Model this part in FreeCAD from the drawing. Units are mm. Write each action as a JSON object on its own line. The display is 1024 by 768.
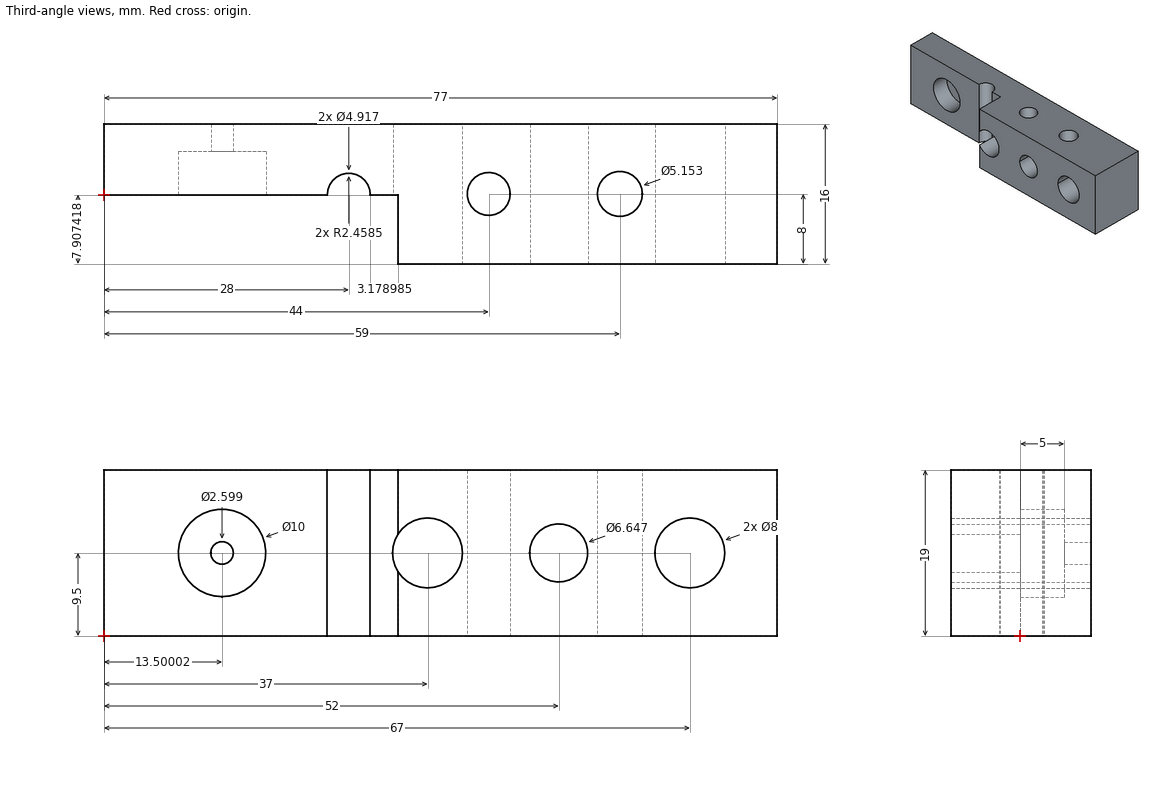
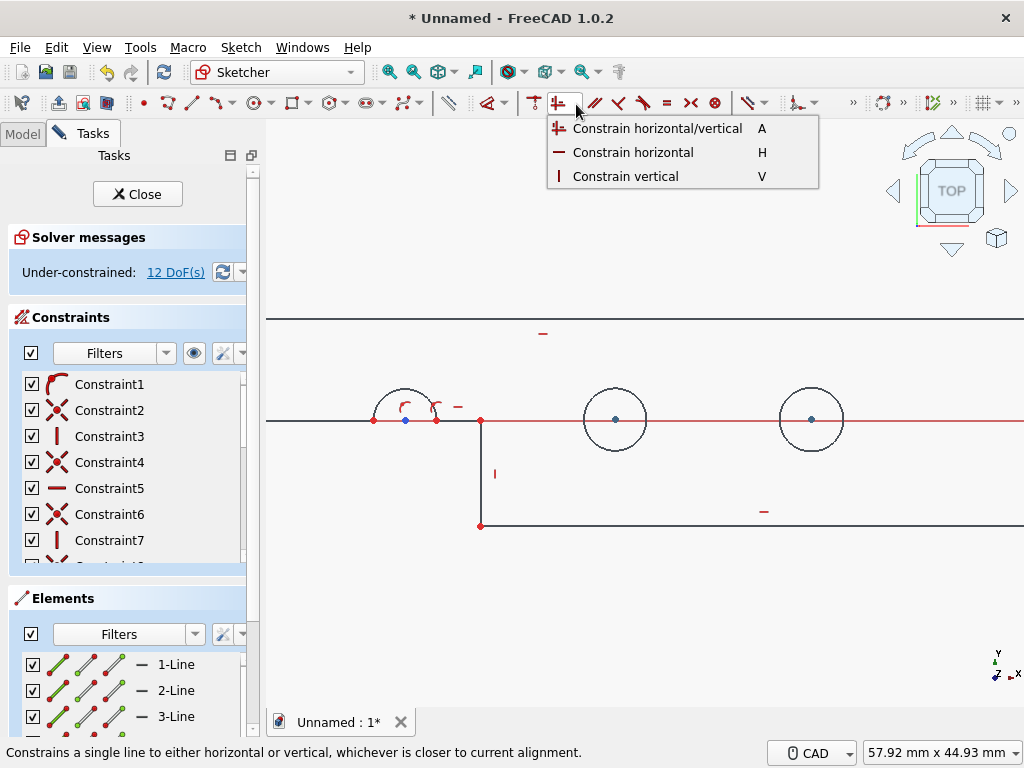
{"action": "left_click", "coordinate": [683, 152]}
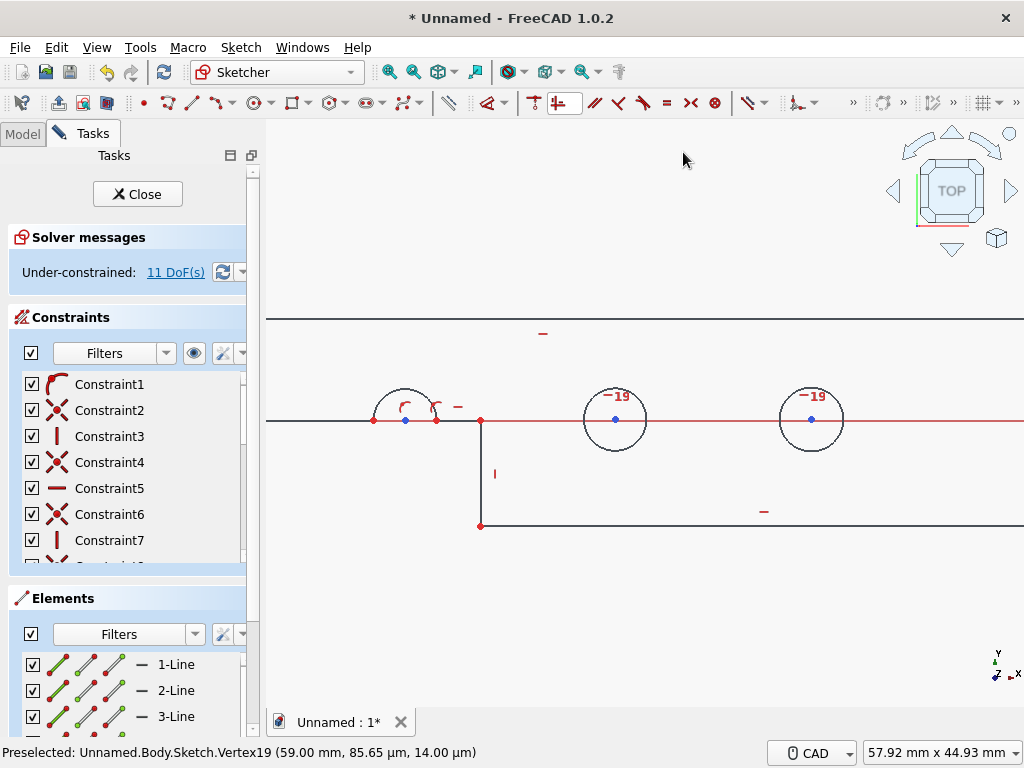
{"action": "left_click", "coordinate": [488, 104]}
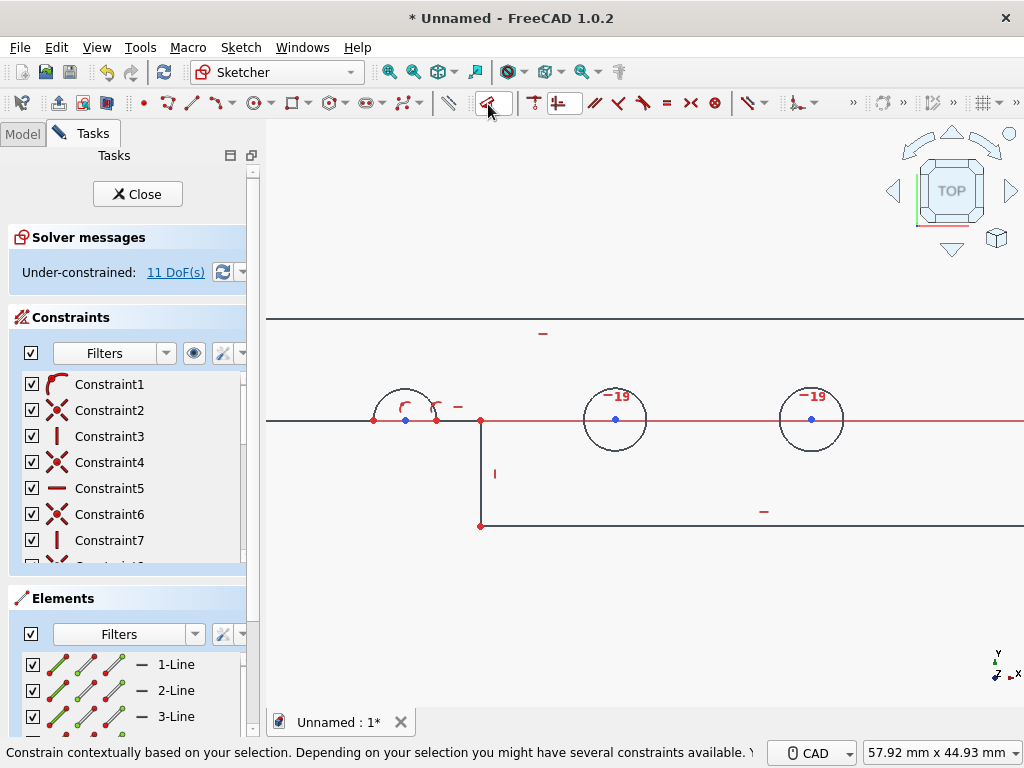
{"action": "scroll", "coordinate": [424, 395], "scroll_direction": "up", "scroll_amount": 2}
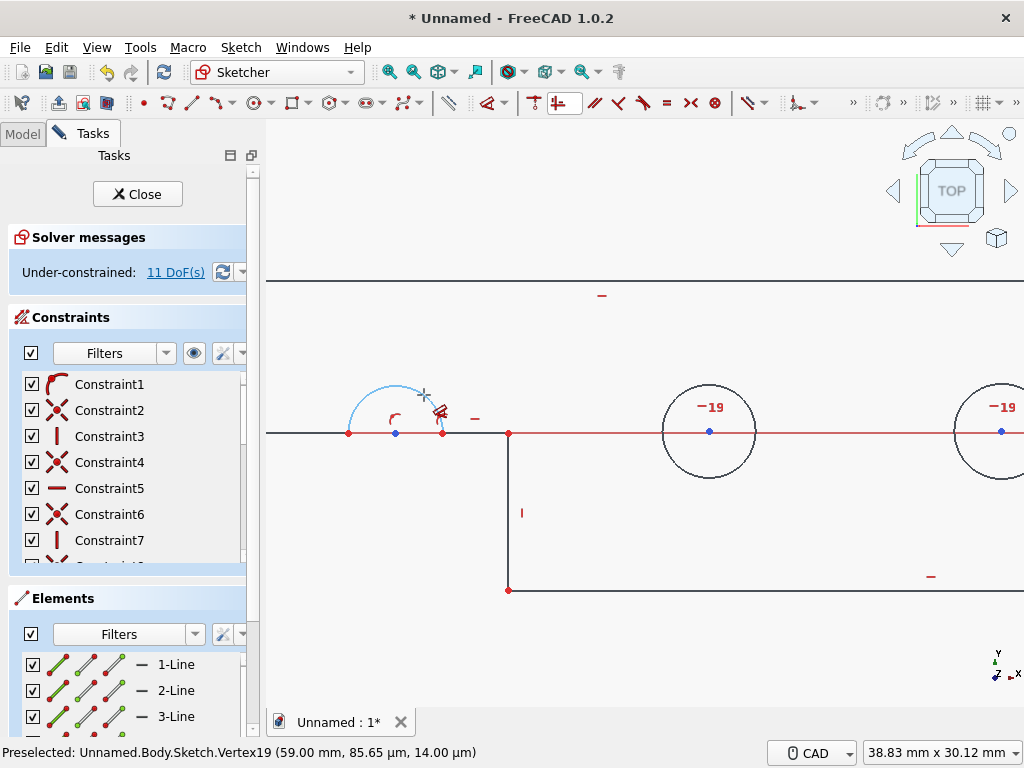
{"action": "left_click", "coordinate": [423, 395]}
{"action": "left_click", "coordinate": [442, 369]}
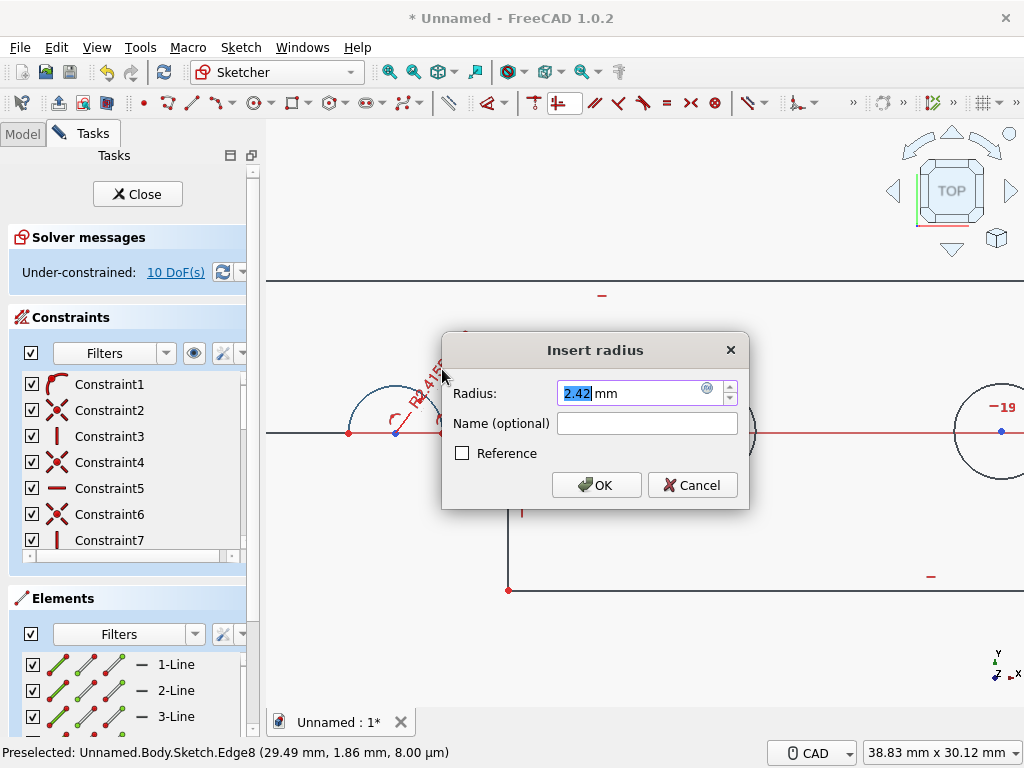
{"action": "type", "text": "2.4585"}
{"action": "key", "text": "Return"}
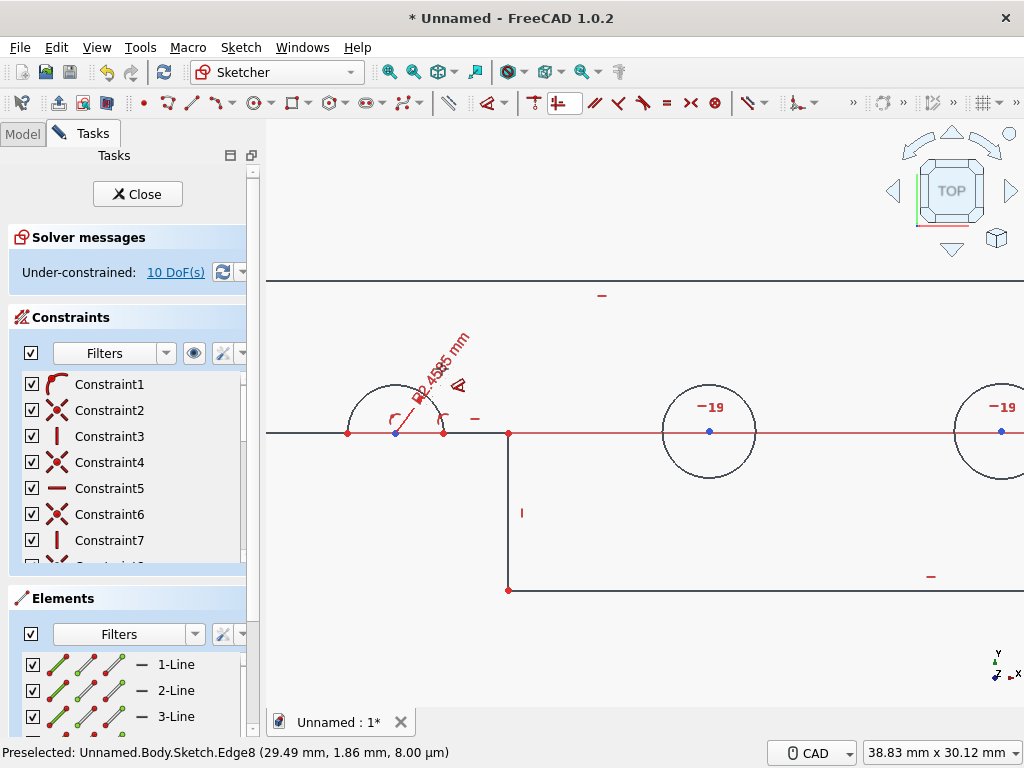
{"action": "left_click", "coordinate": [742, 398]}
{"action": "left_click", "coordinate": [764, 375]}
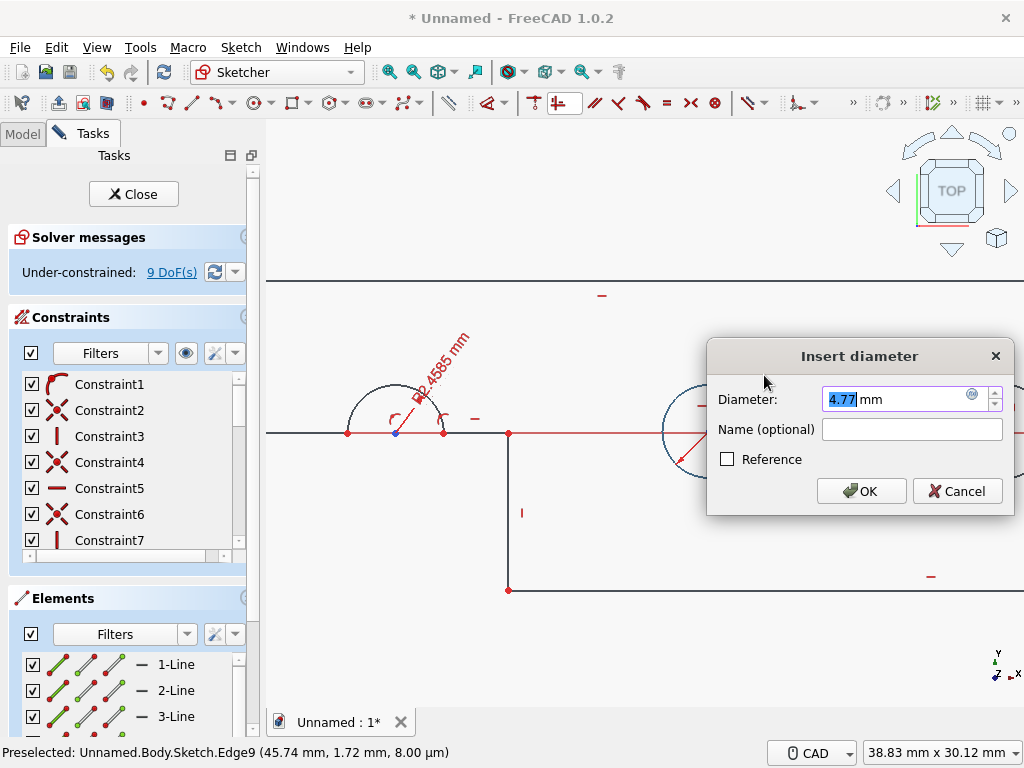
{"action": "type", "text": "4.917"}
{"action": "key", "text": "Return"}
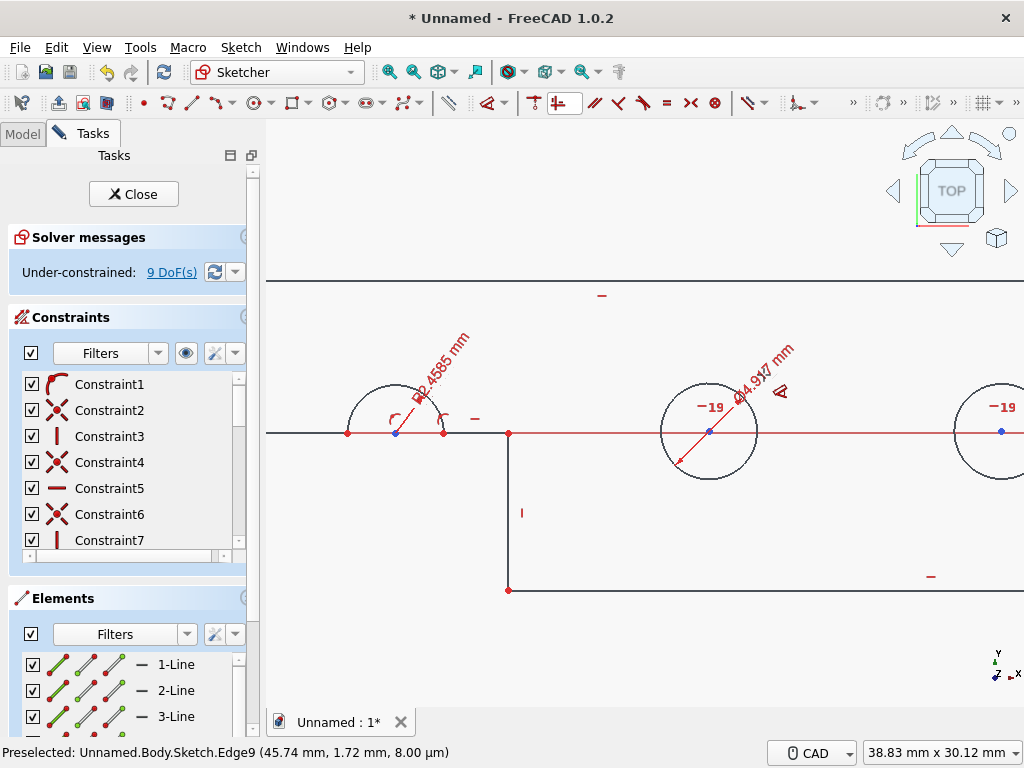
{"action": "scroll", "coordinate": [568, 407], "scroll_direction": "down", "scroll_amount": 7}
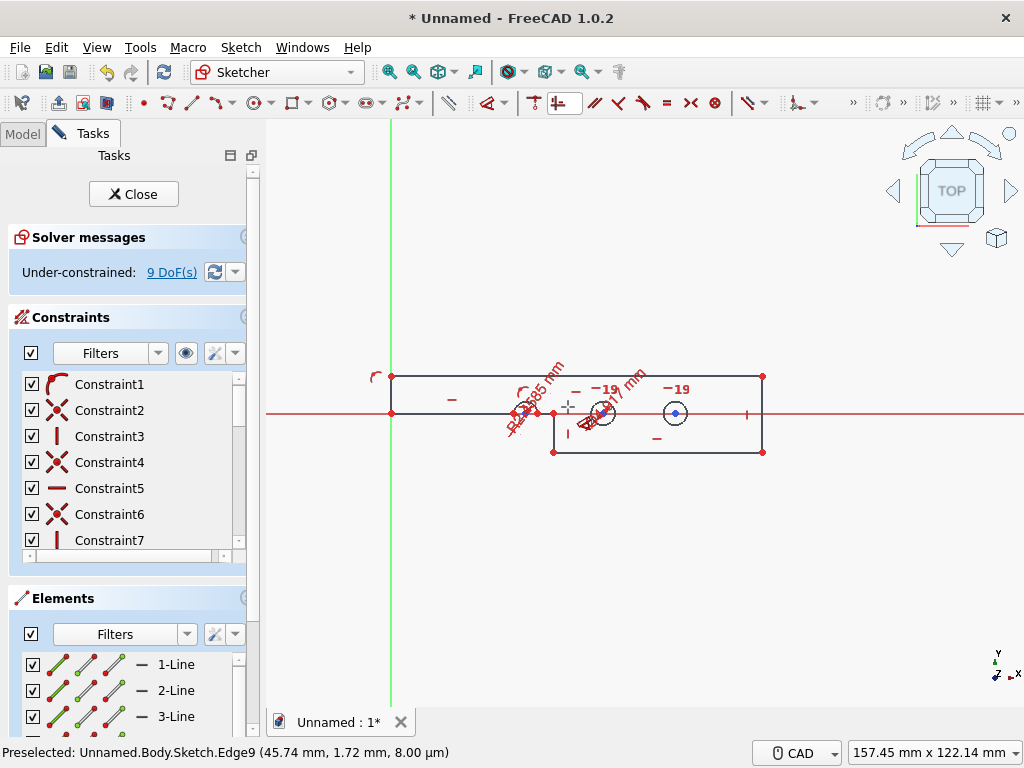
{"action": "scroll", "coordinate": [684, 405], "scroll_direction": "up", "scroll_amount": 3}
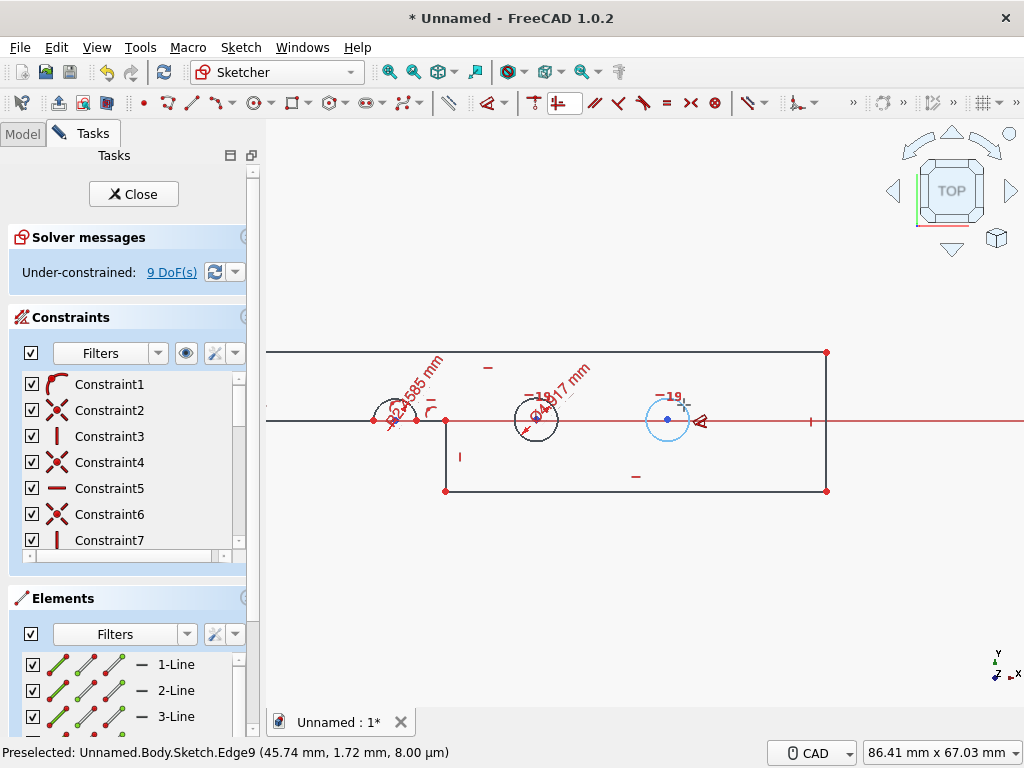
{"action": "left_click", "coordinate": [683, 405]}
{"action": "left_click", "coordinate": [706, 383]}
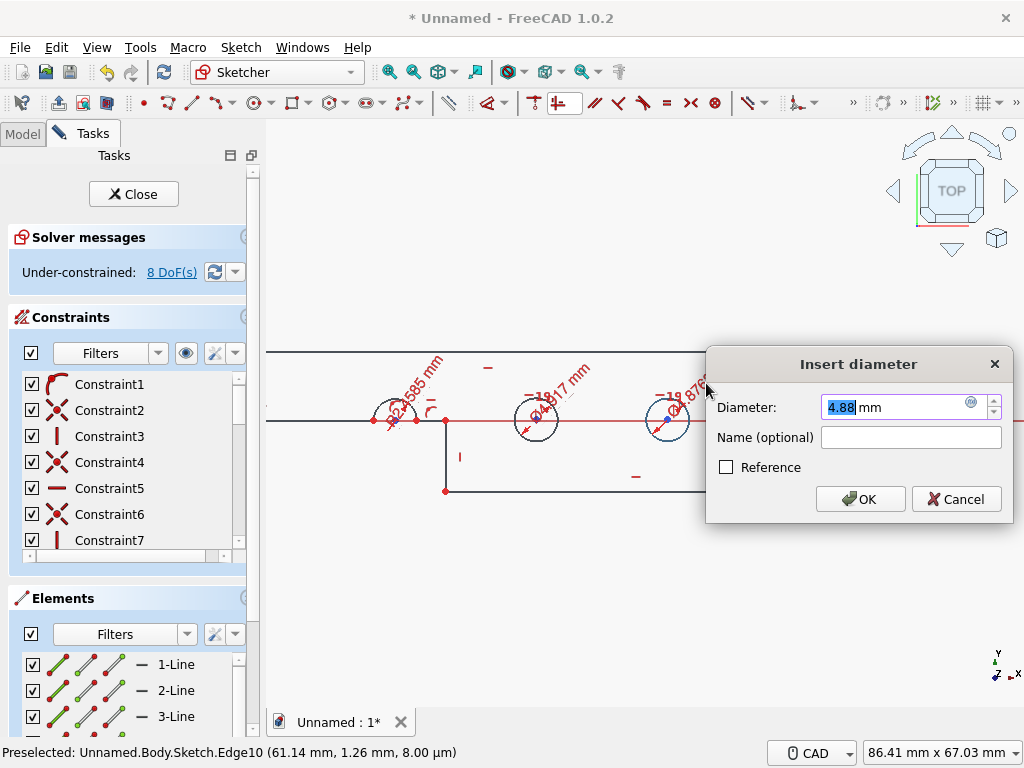
{"action": "type", "text": "5.153"}
{"action": "key", "text": "Return"}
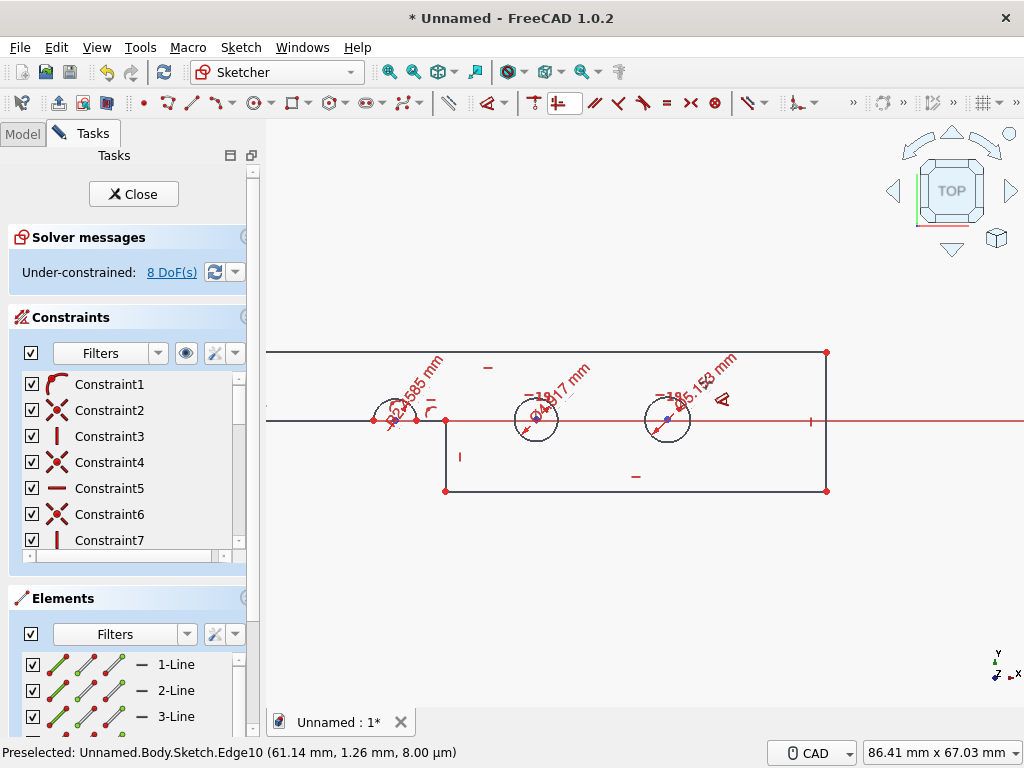
{"action": "left_click", "coordinate": [826, 450]}
{"action": "left_click", "coordinate": [792, 390]}